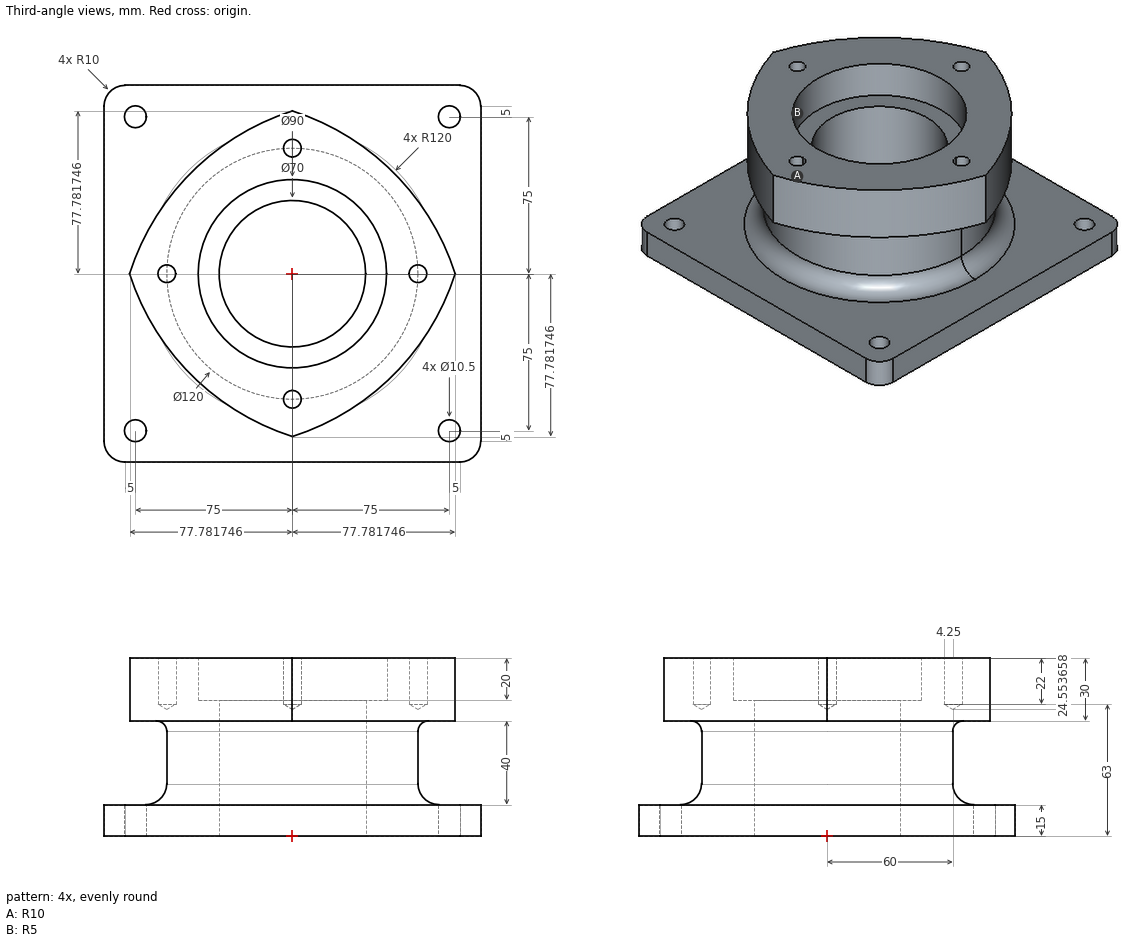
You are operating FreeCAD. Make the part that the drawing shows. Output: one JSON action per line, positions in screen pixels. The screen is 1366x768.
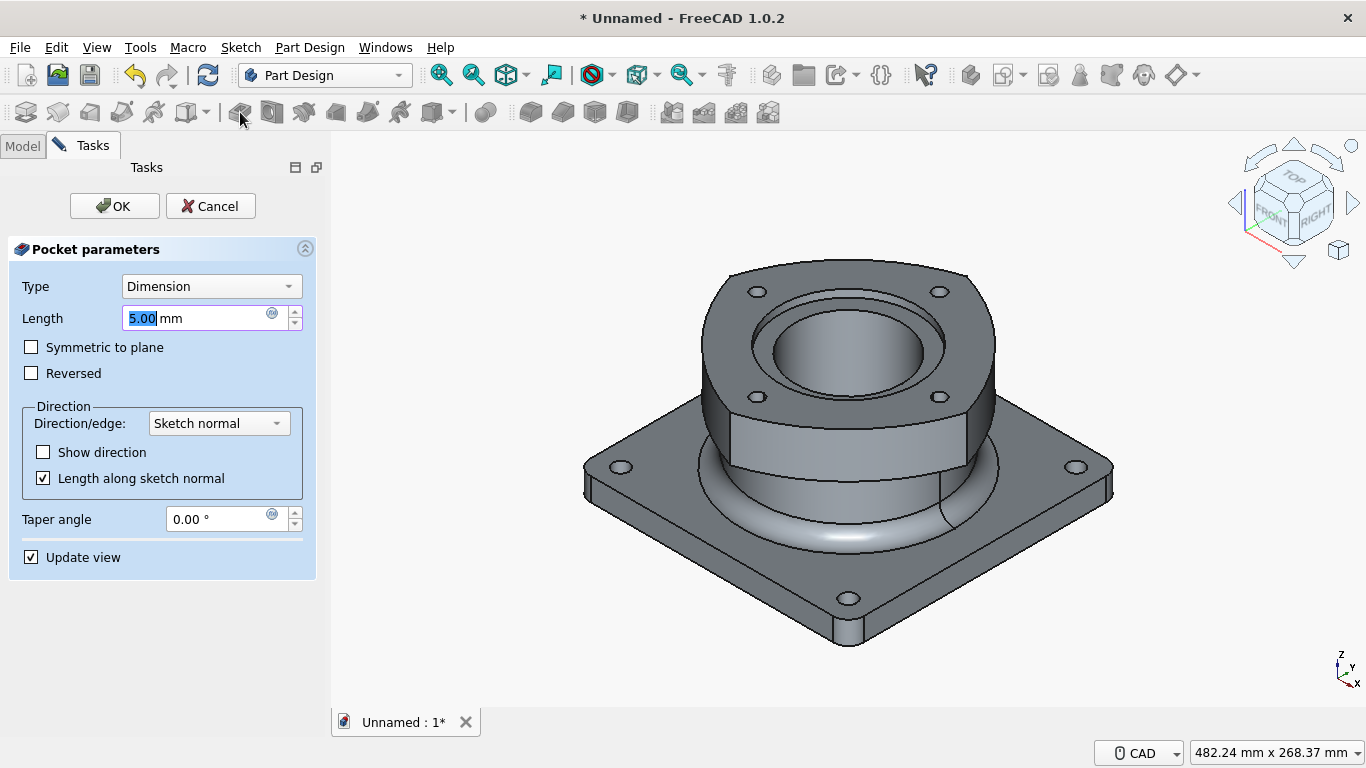
{"action": "type", "text": "20"}
{"action": "key", "text": "Tab"}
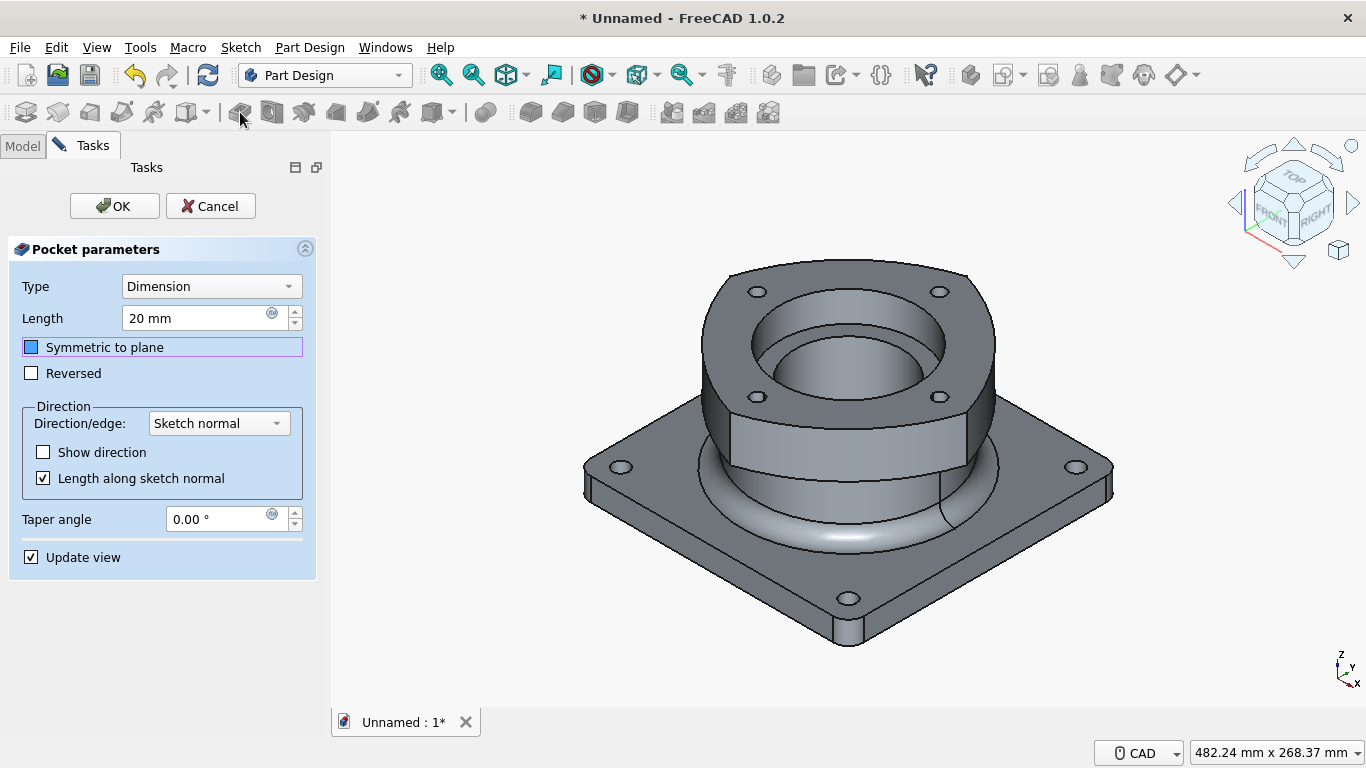
{"action": "left_click", "coordinate": [115, 206]}